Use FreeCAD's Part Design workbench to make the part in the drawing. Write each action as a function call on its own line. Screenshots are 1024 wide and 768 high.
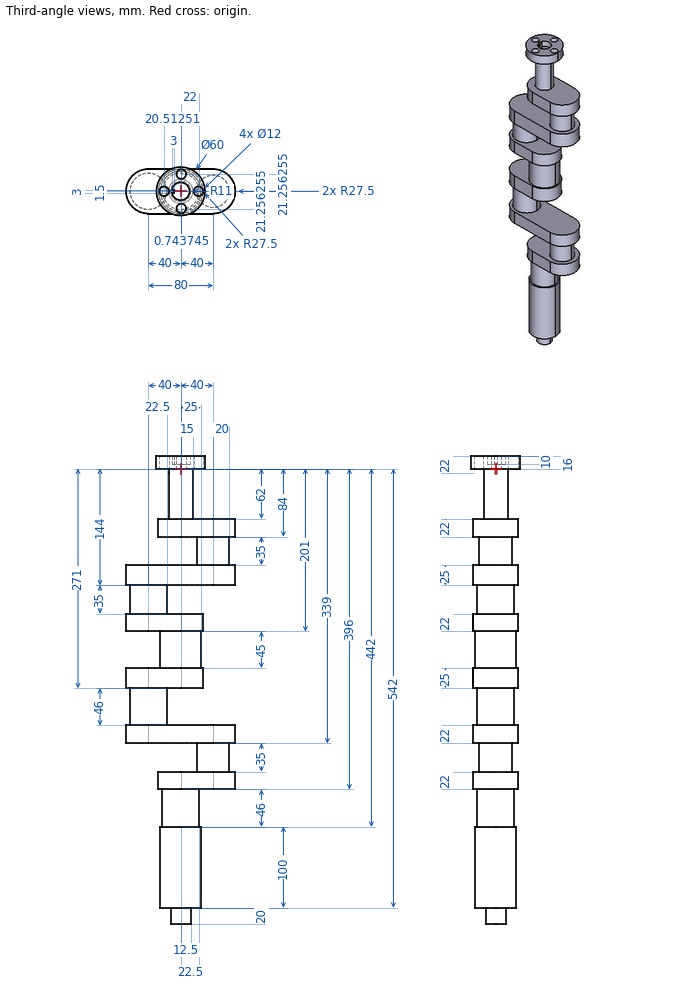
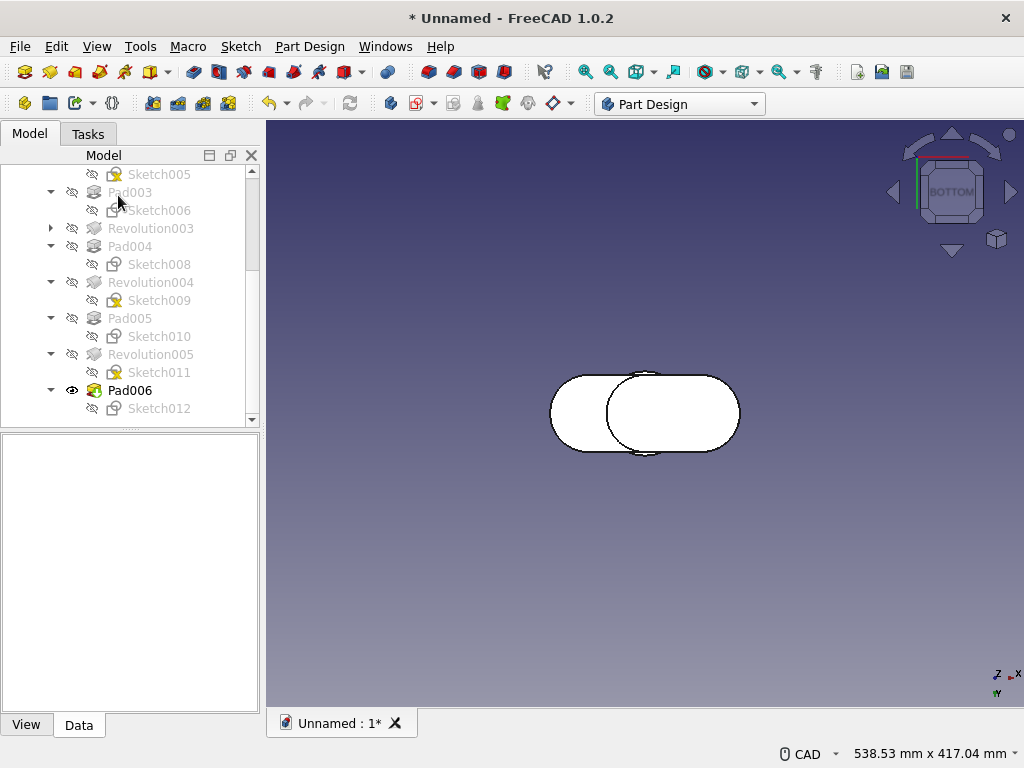
click(586, 72)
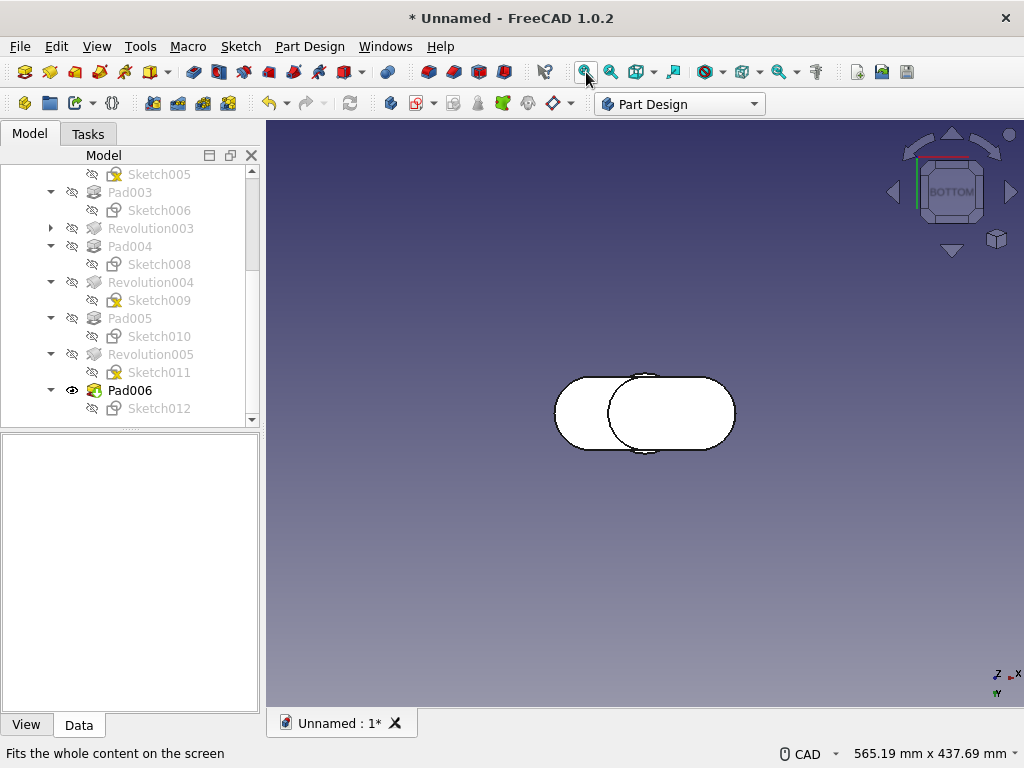
click(416, 104)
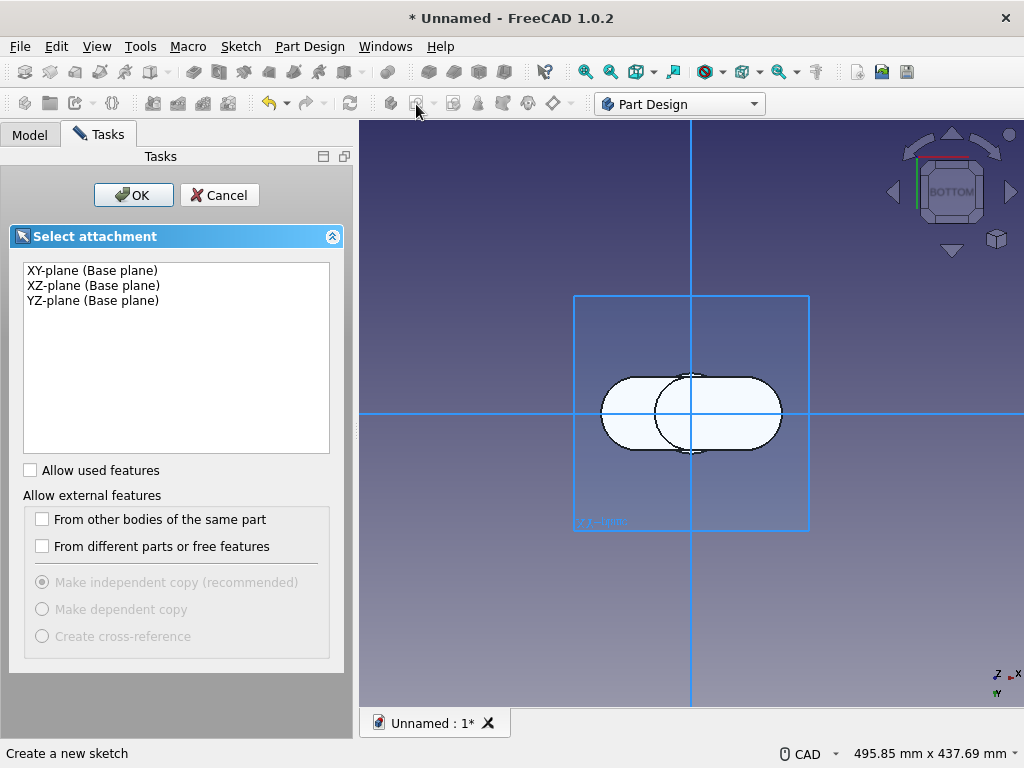
click(84, 286)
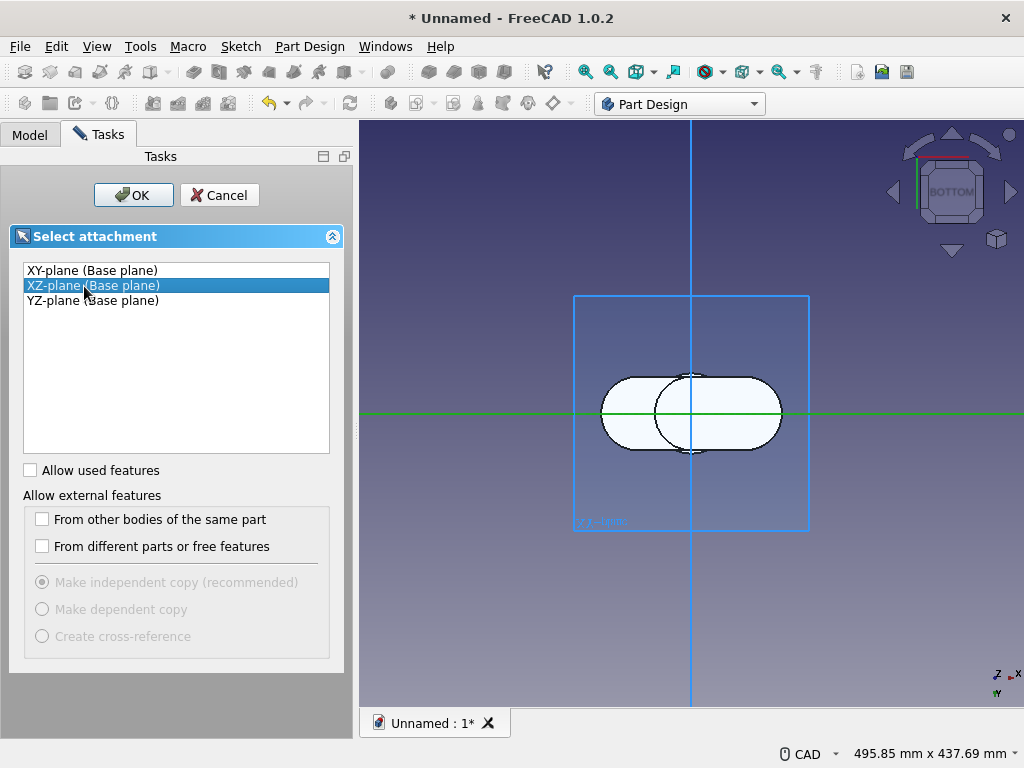
click(134, 195)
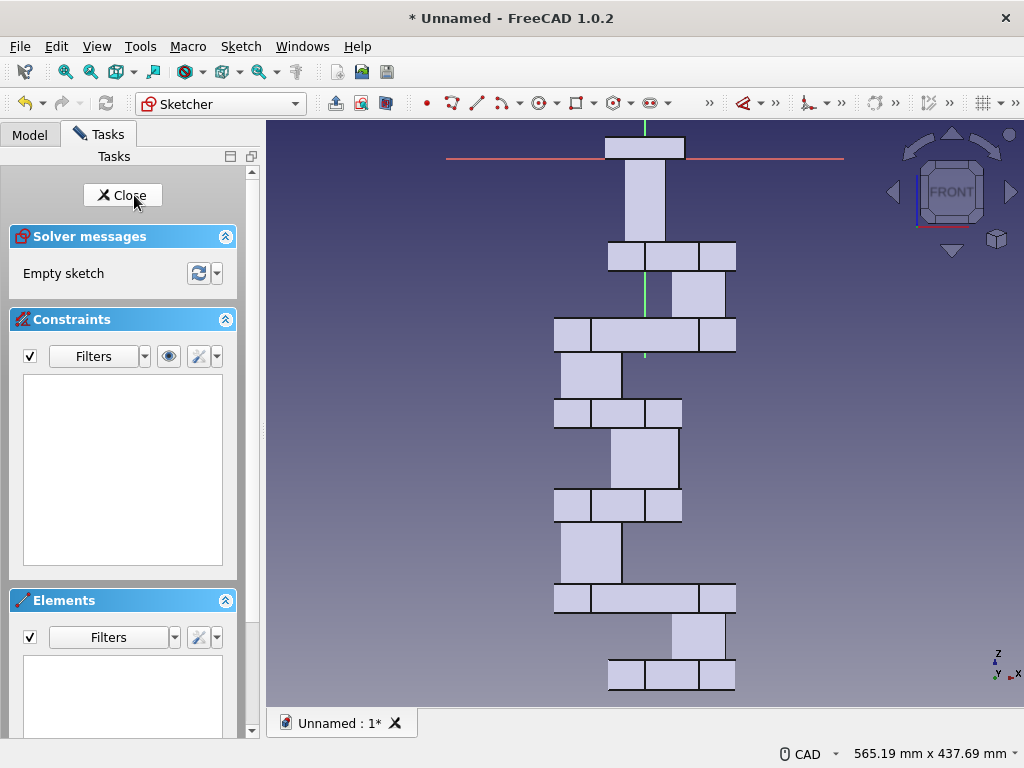
key(q)
key(s)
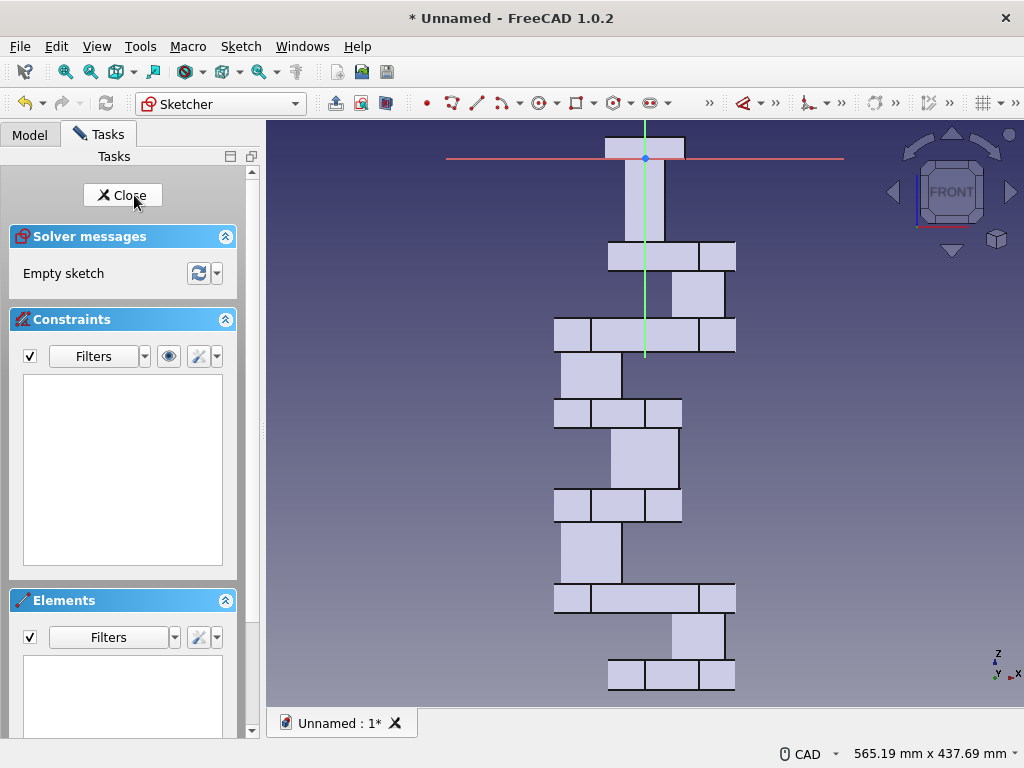
scroll(576, 414, down, 5)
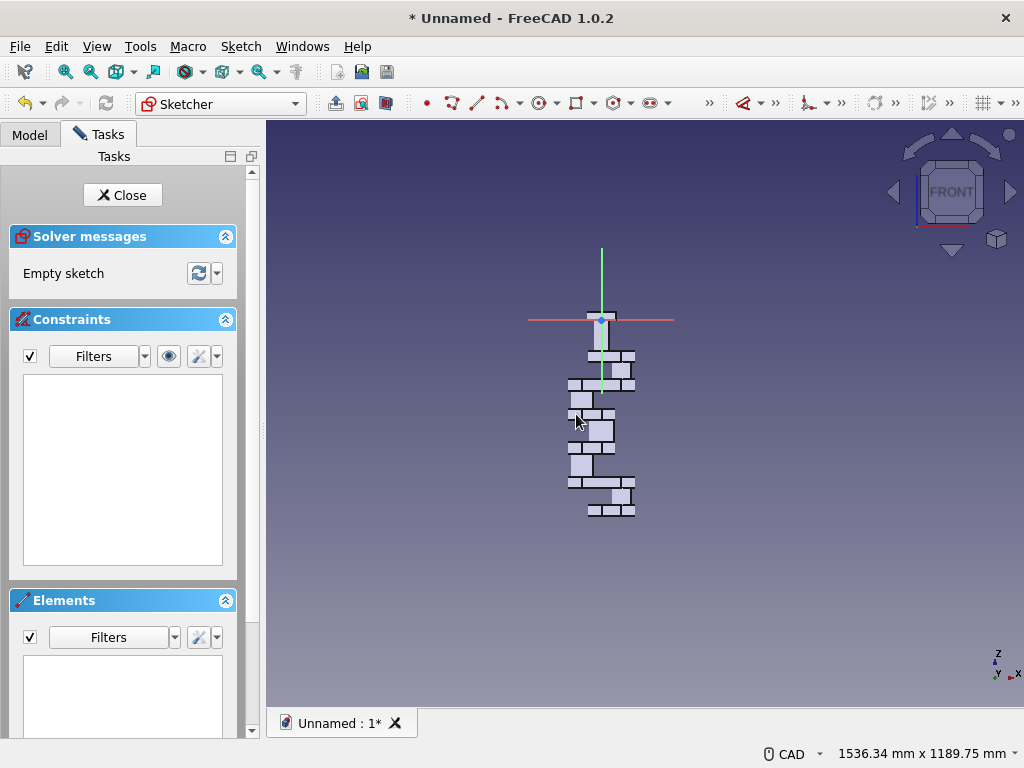
scroll(609, 534, up, 14)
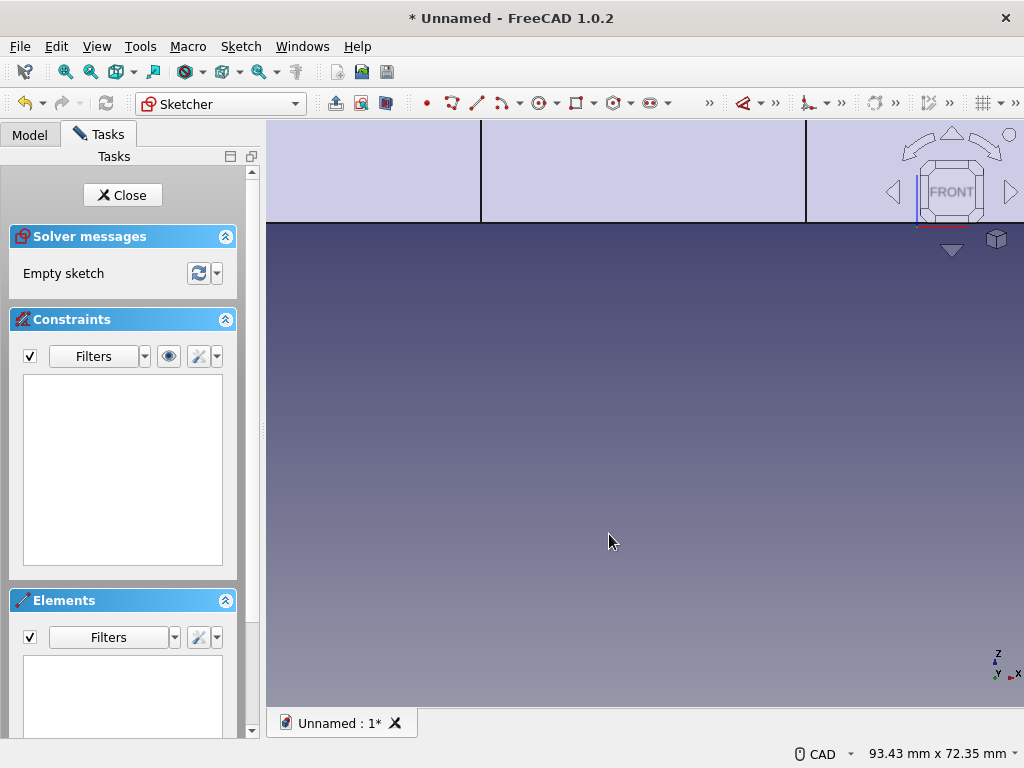
key(g)
key(r)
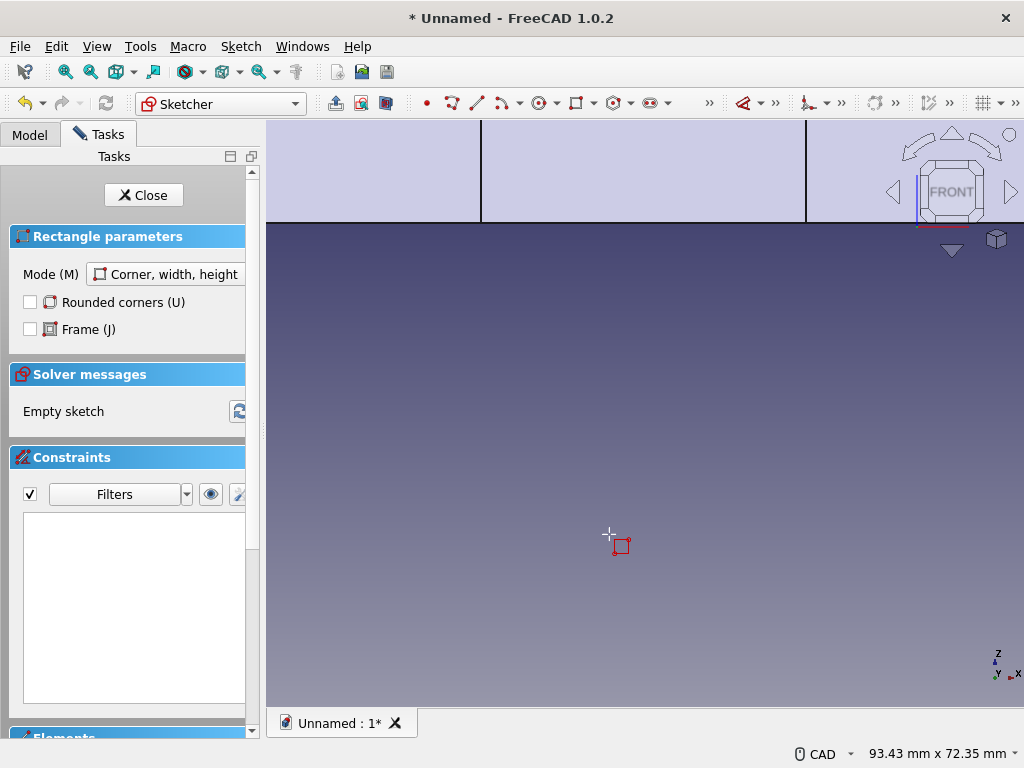
click(481, 223)
move(664, 597)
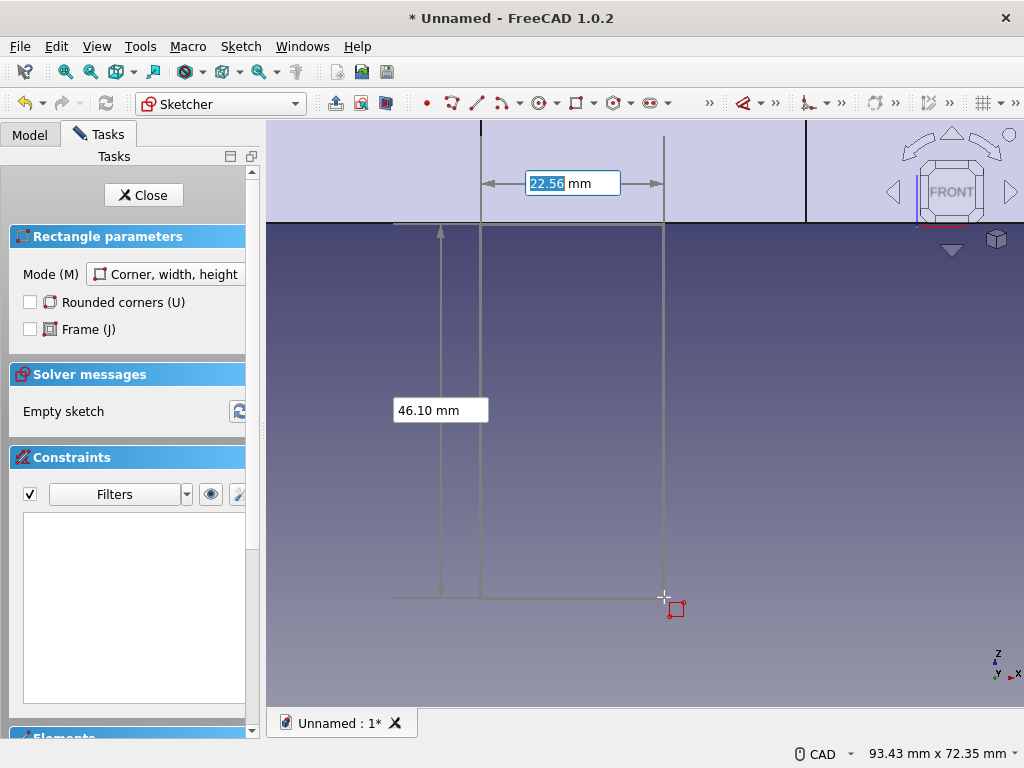
text(22.5)
key(Tab)
text(46)
key(Return)
key(Escape)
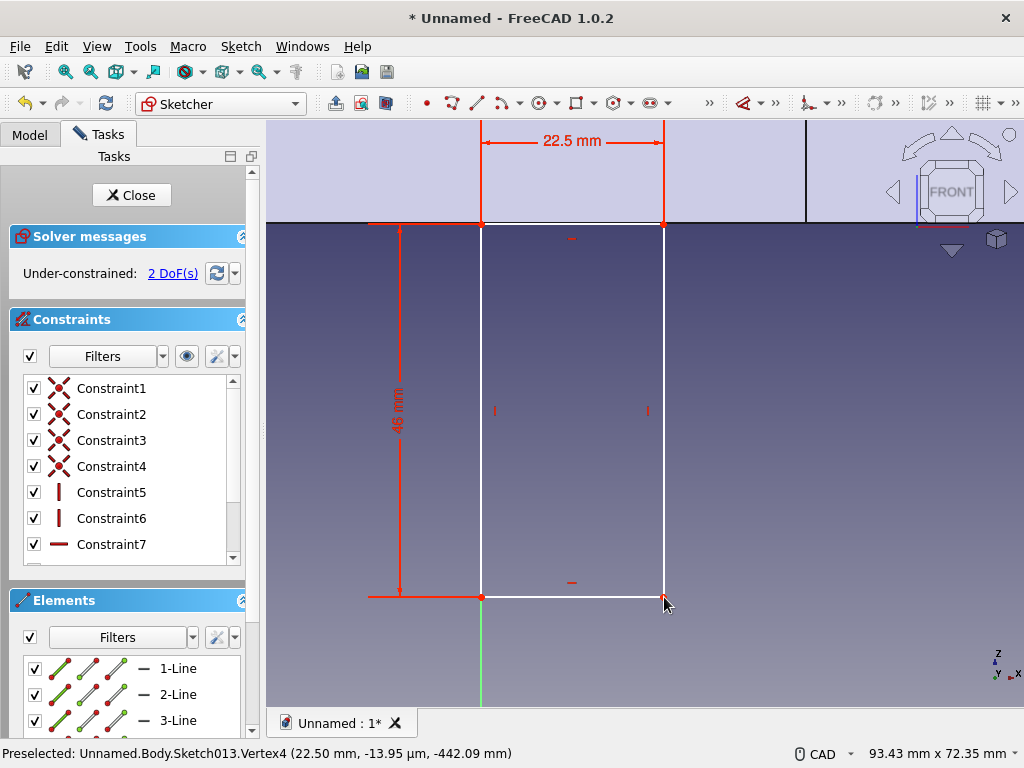
click(481, 224)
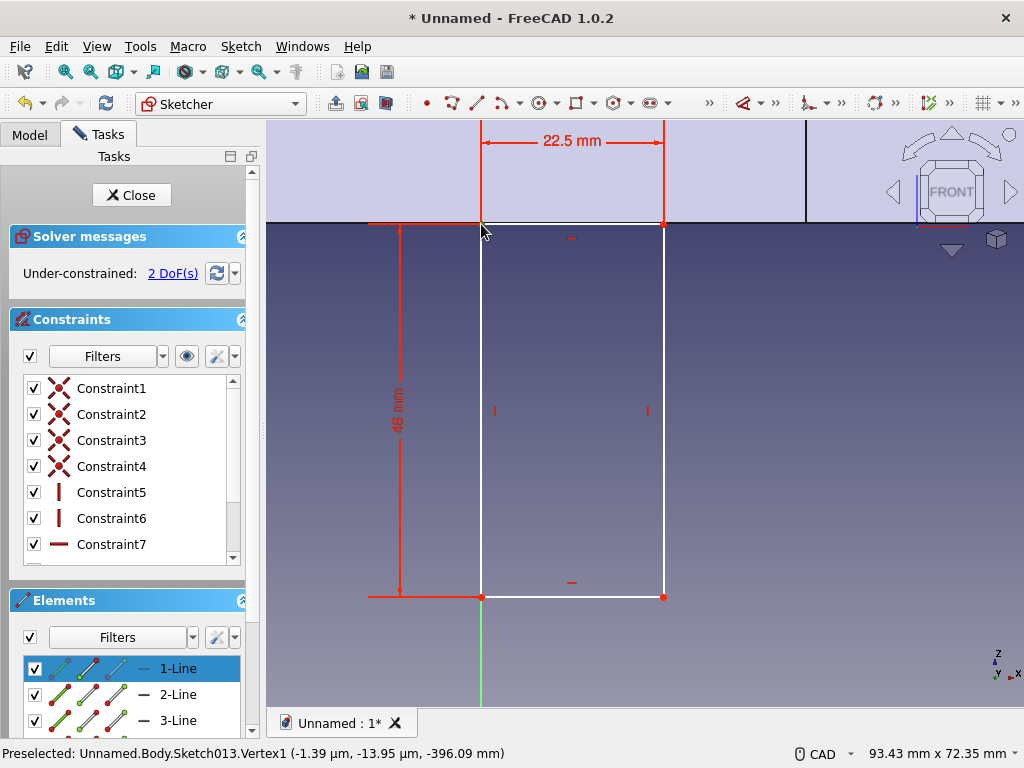
click(481, 641)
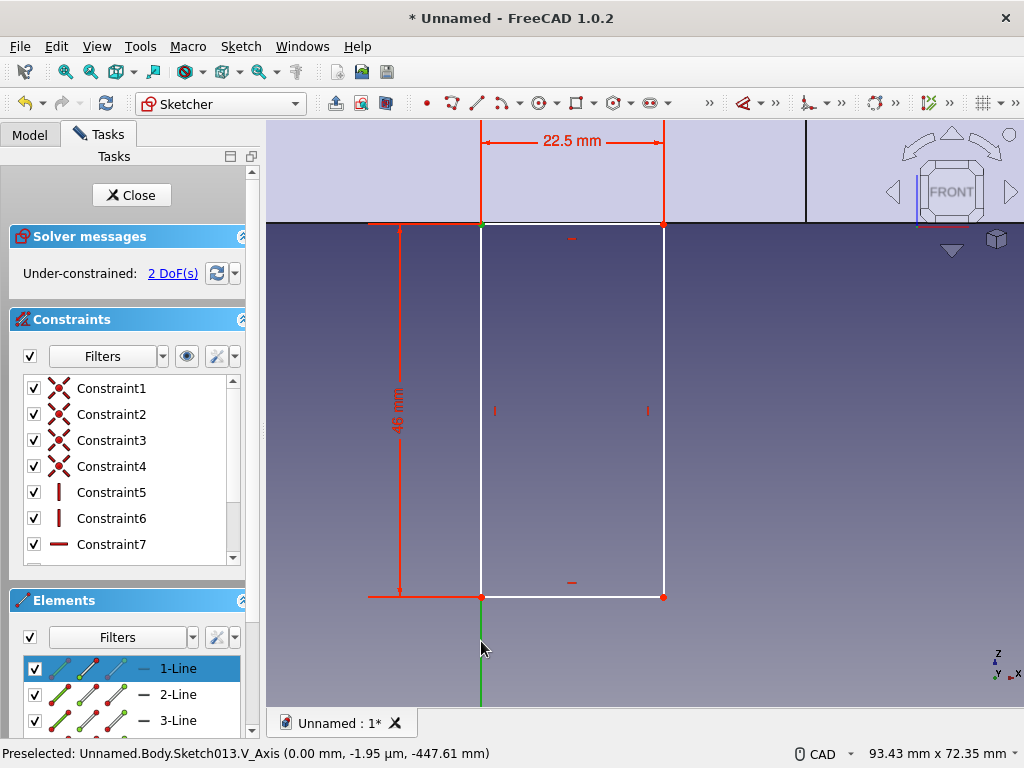
key(c)